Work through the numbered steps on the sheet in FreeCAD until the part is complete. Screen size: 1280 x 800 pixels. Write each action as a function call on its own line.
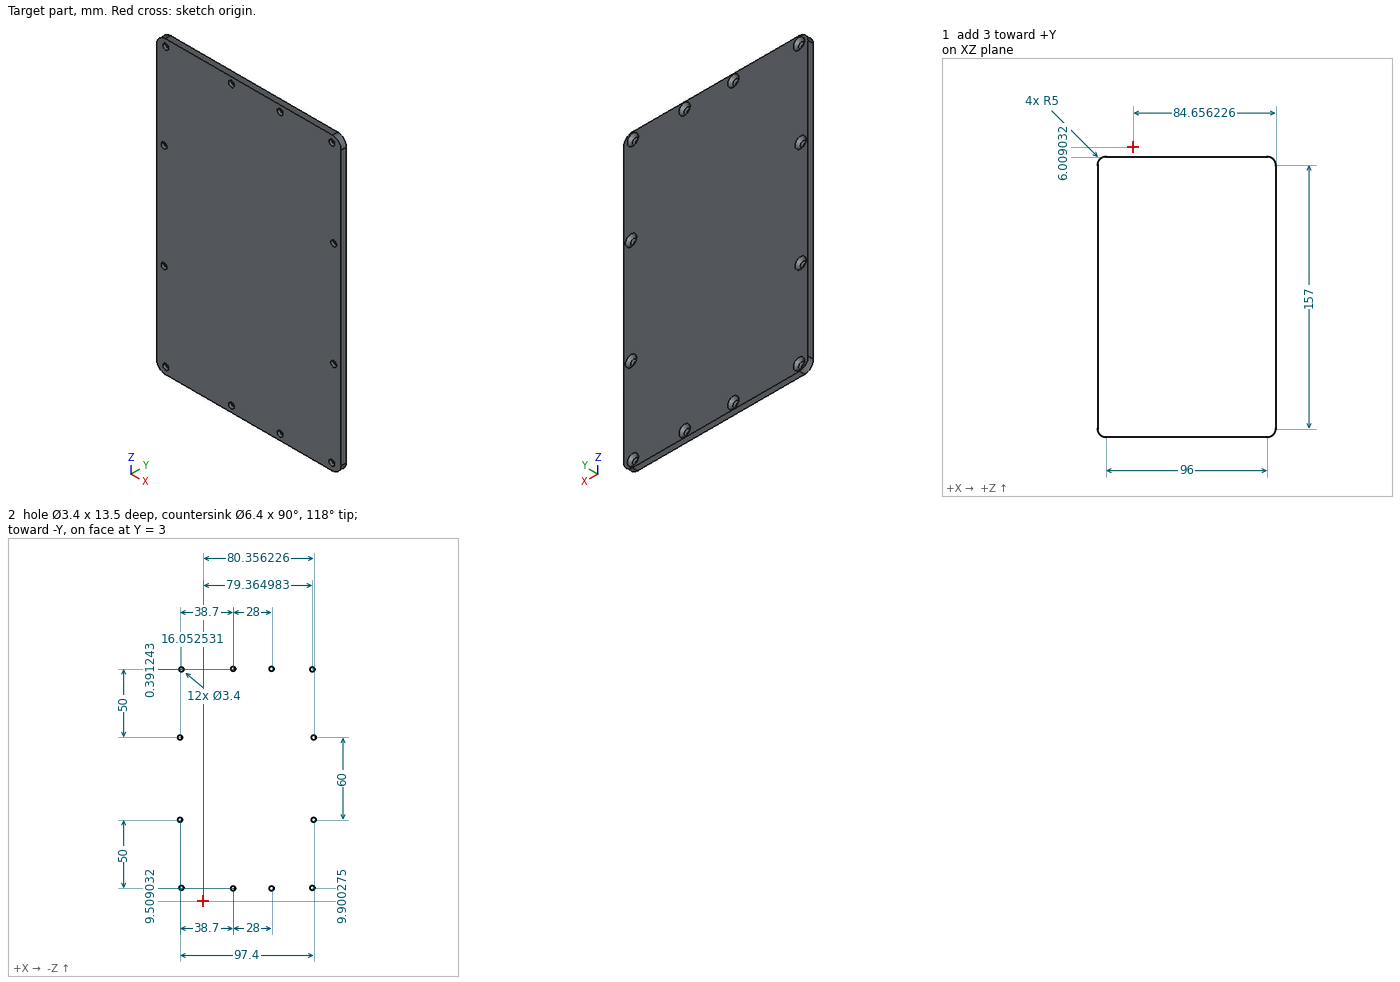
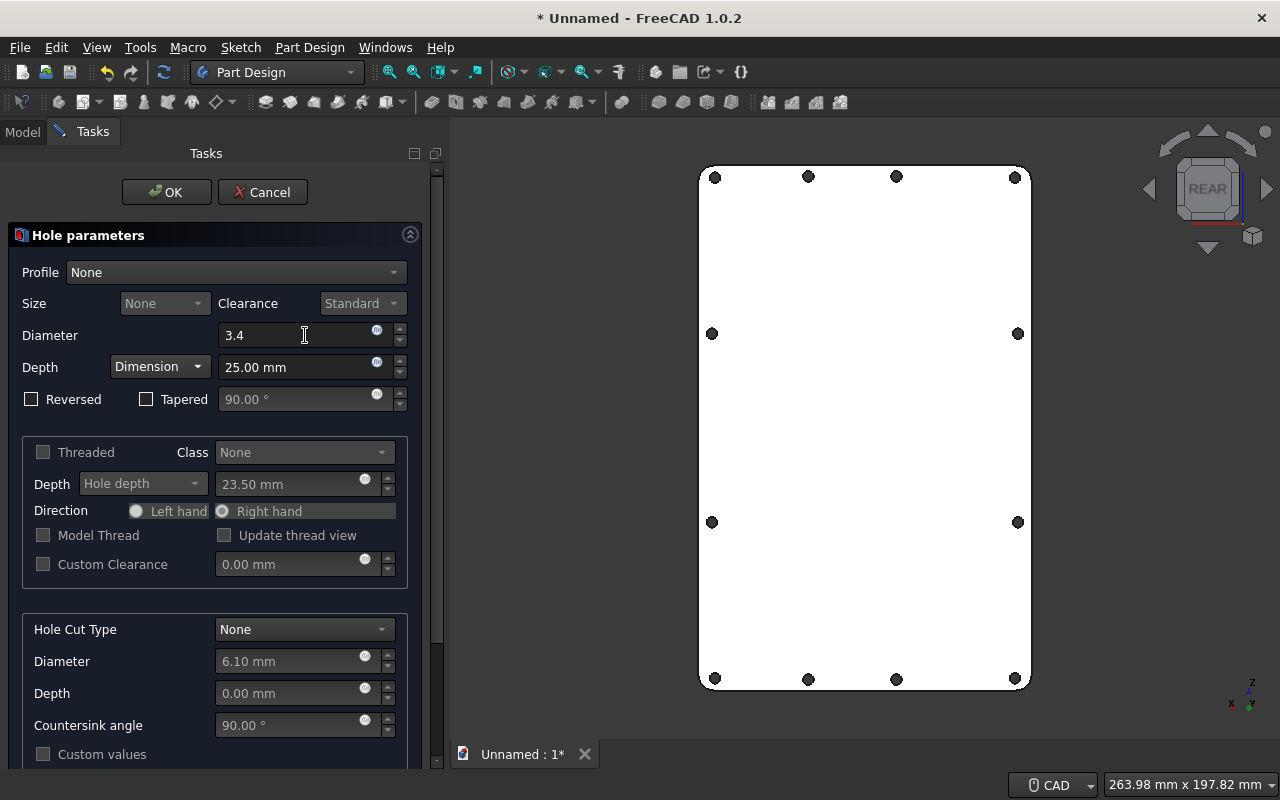
triple_click(305, 367)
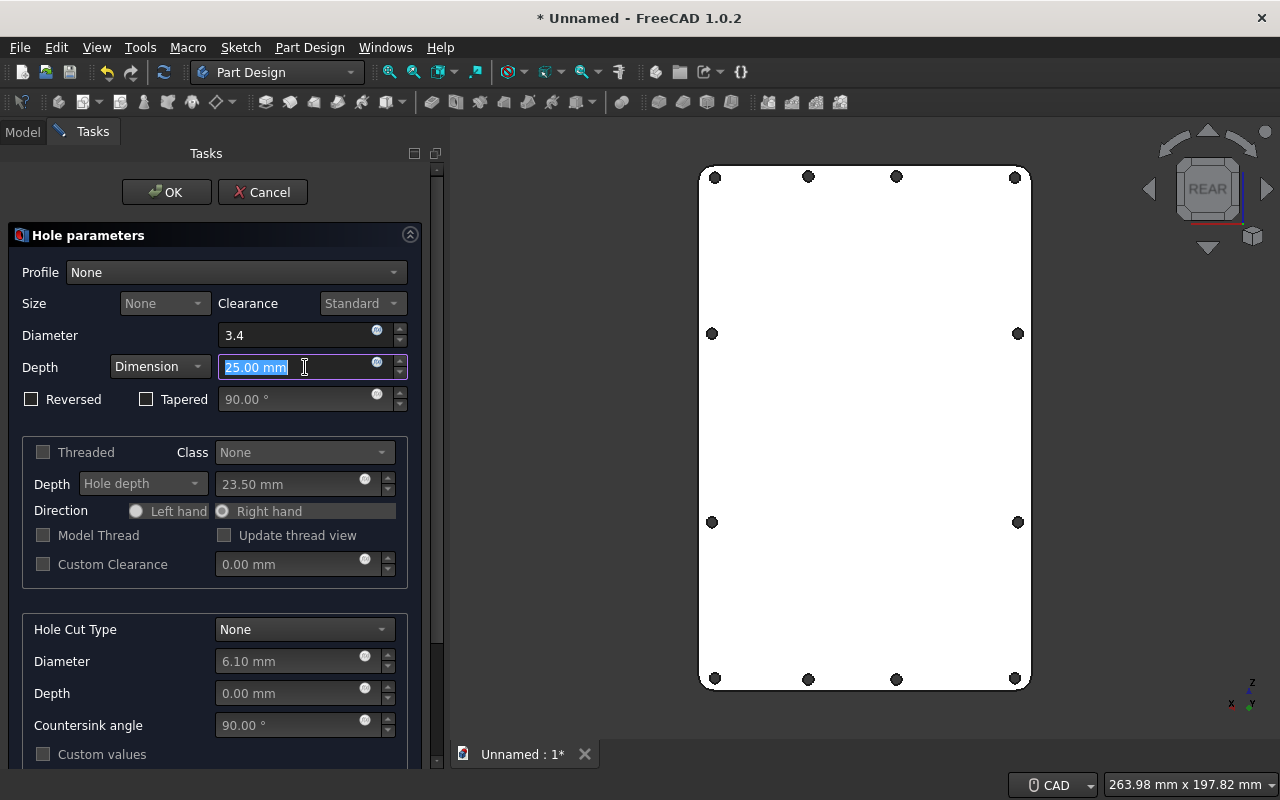
text(13.5)
key(Tab)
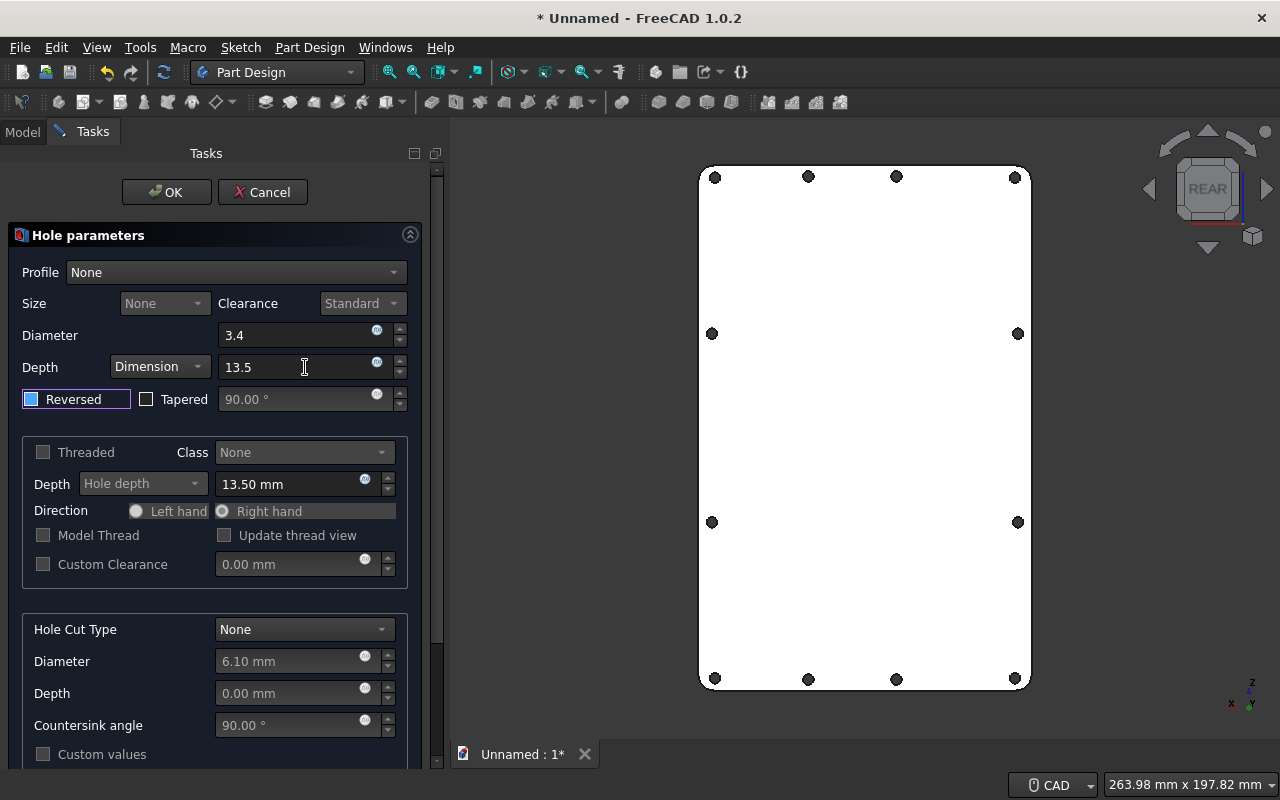
click(306, 630)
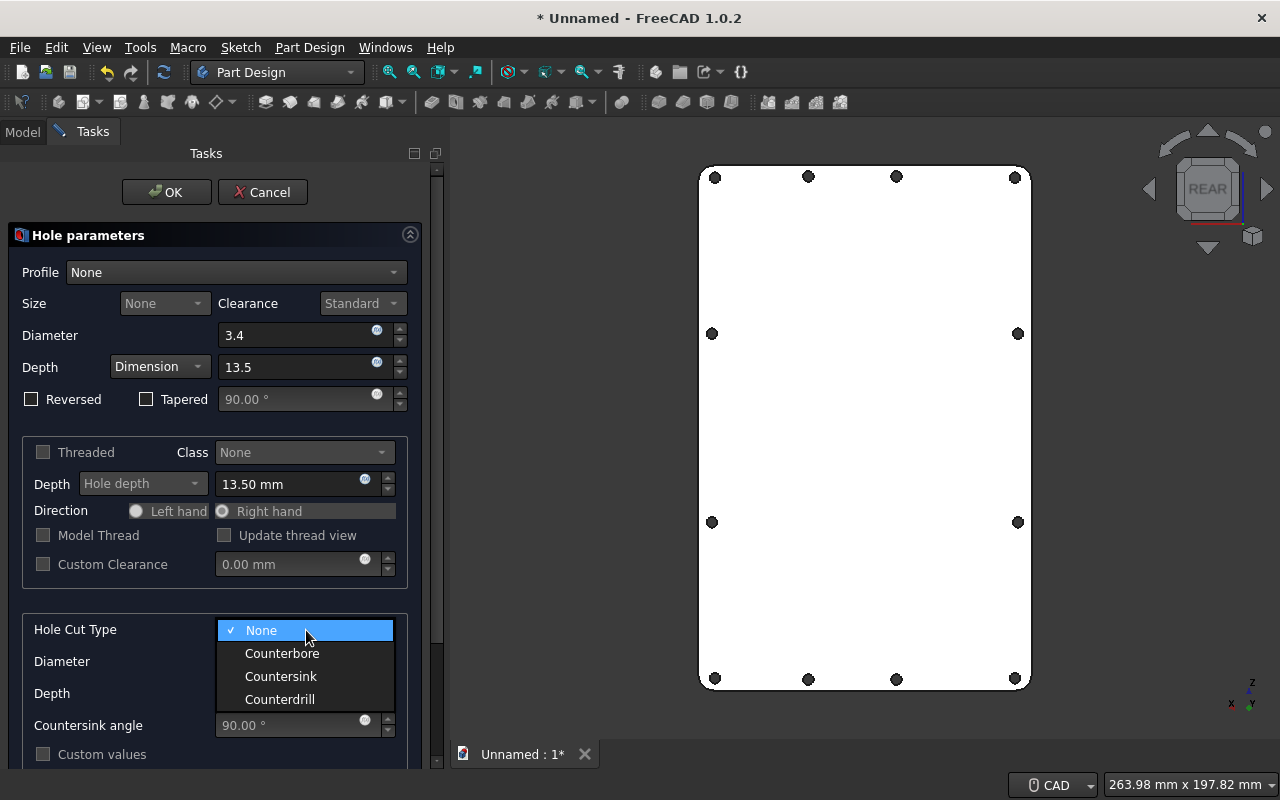
click(304, 676)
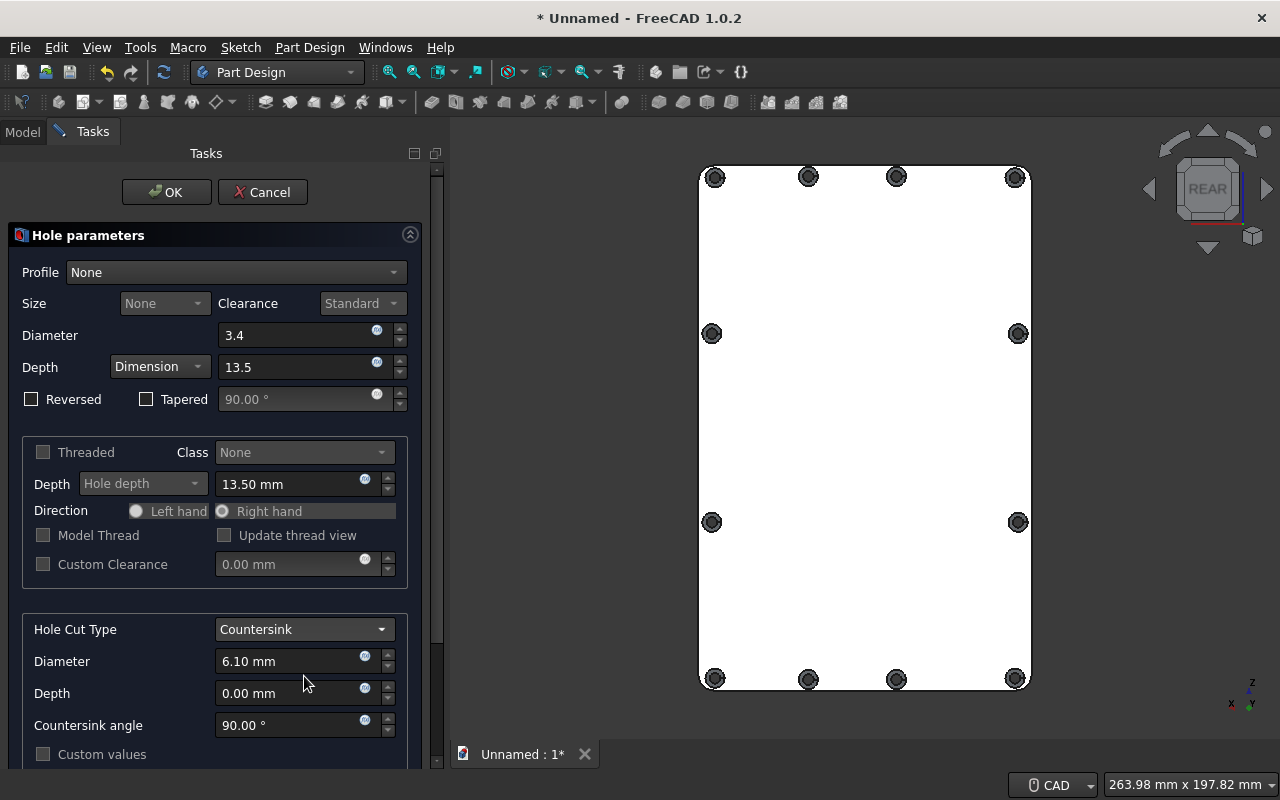
triple_click(298, 661)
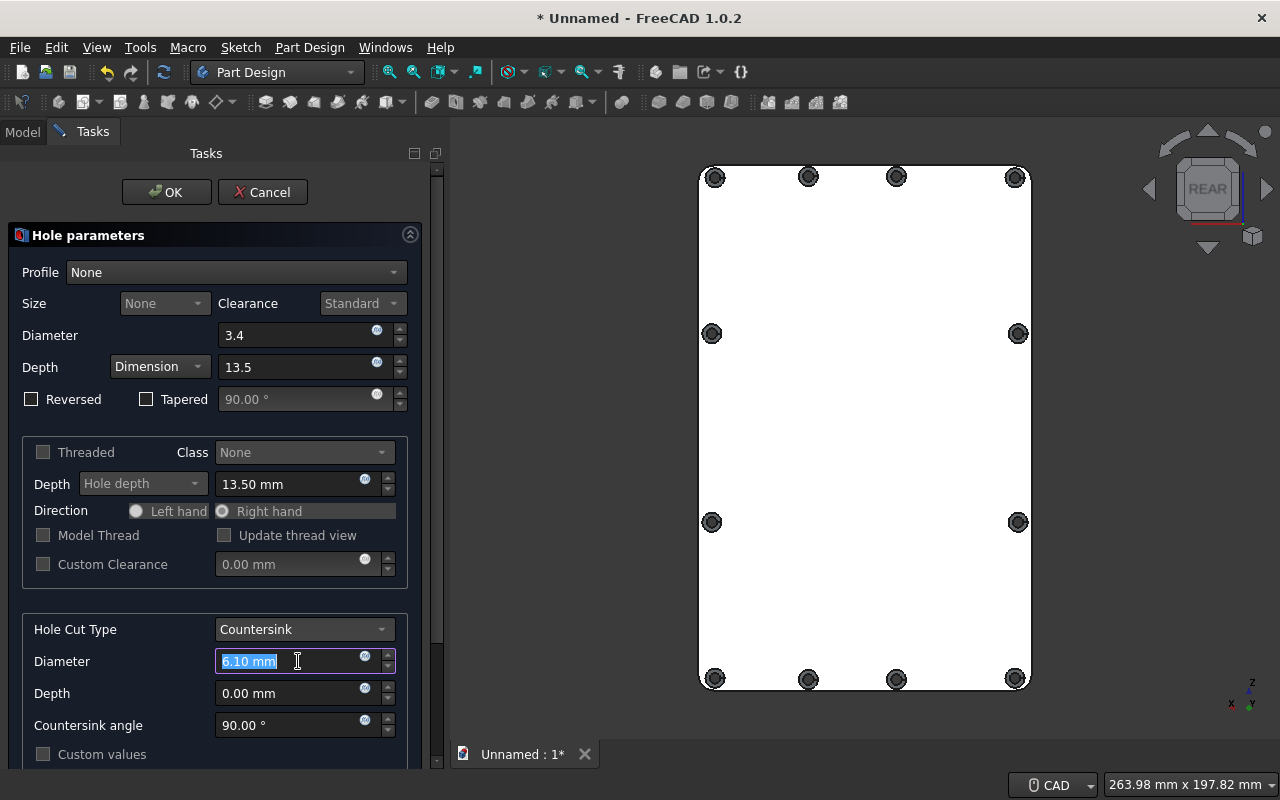
text(6.4)
key(Tab)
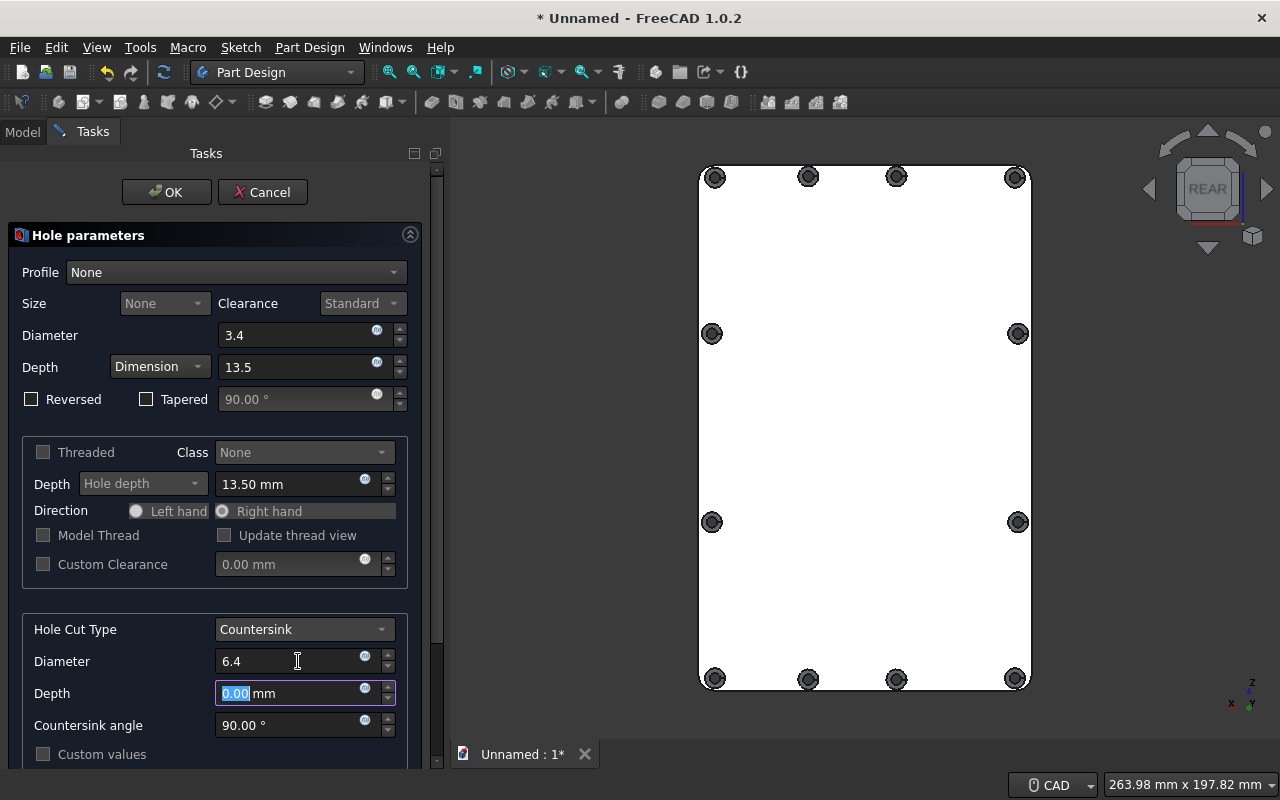
click(167, 192)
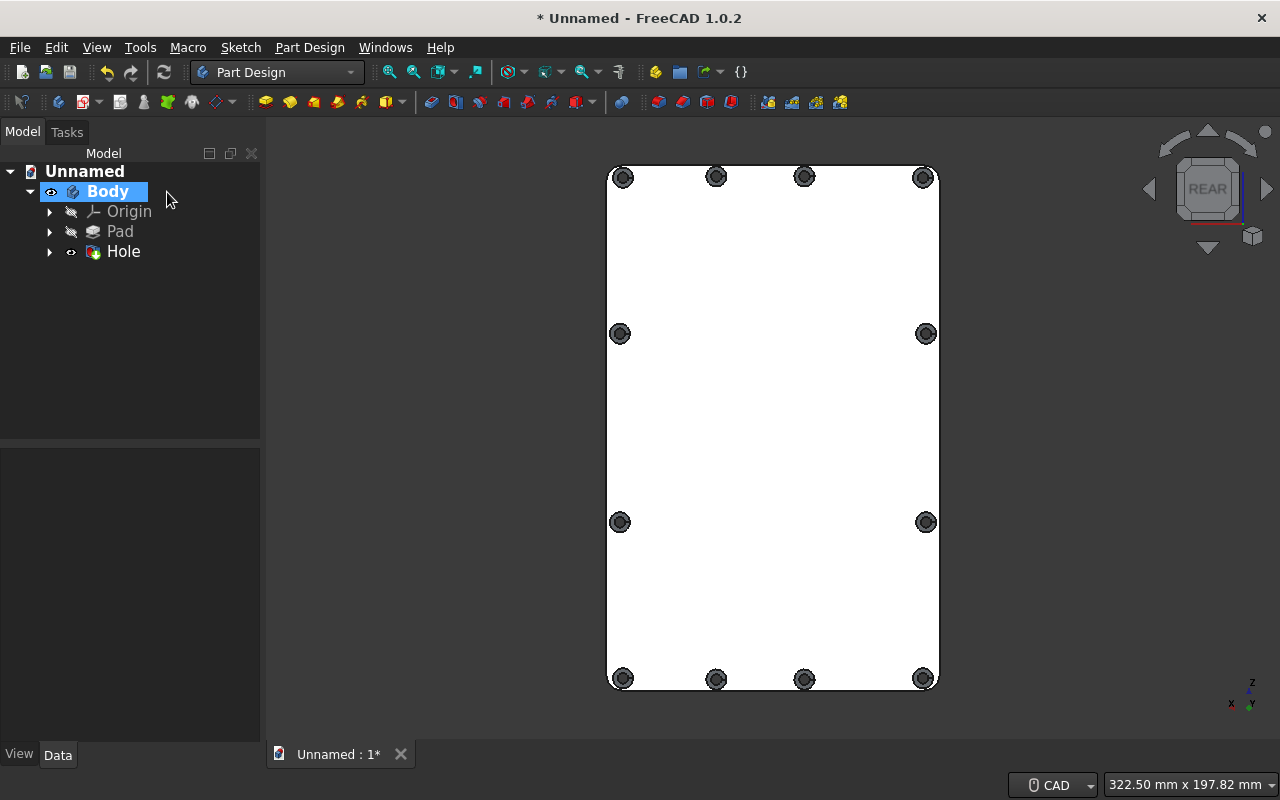
key(0)